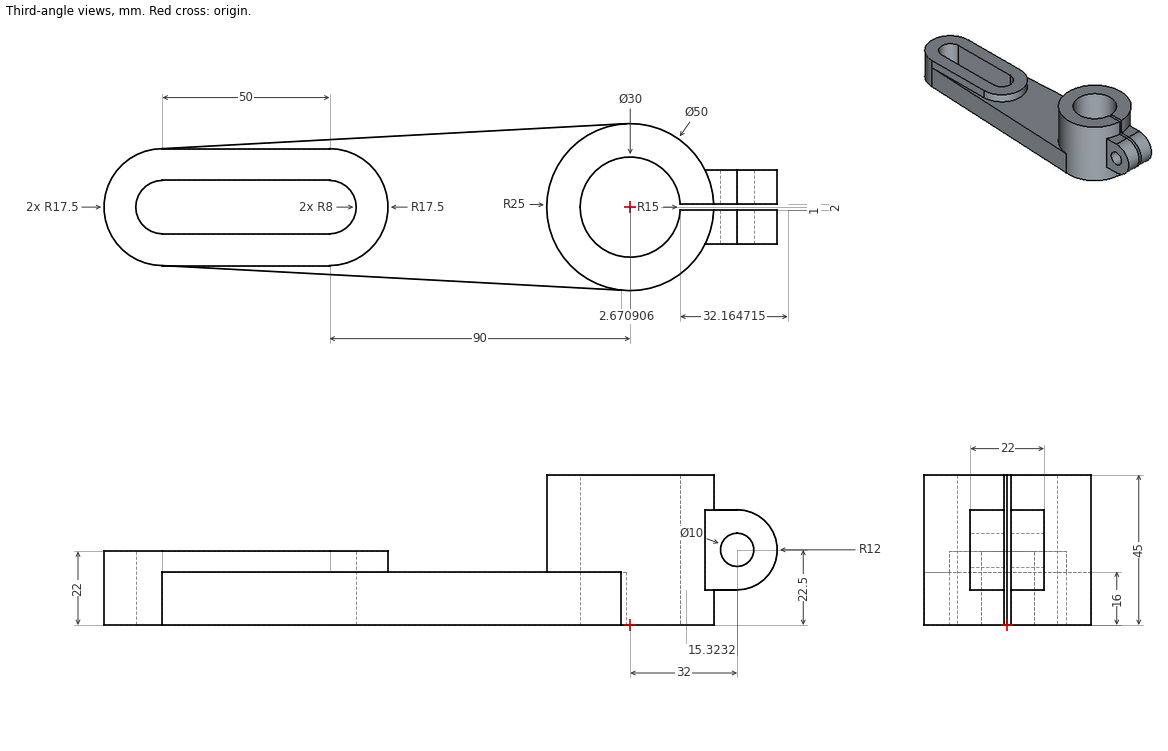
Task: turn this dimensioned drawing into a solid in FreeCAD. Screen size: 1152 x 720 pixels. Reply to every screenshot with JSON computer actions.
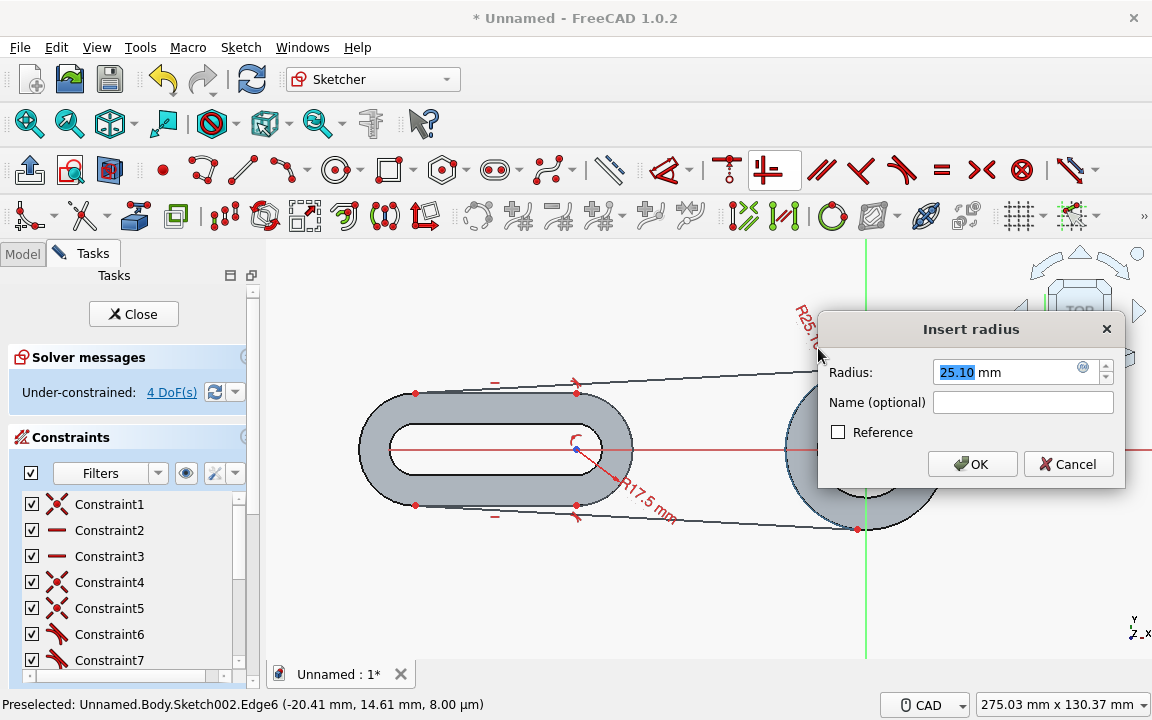
{"action": "type", "text": "25"}
{"action": "key", "text": "Return"}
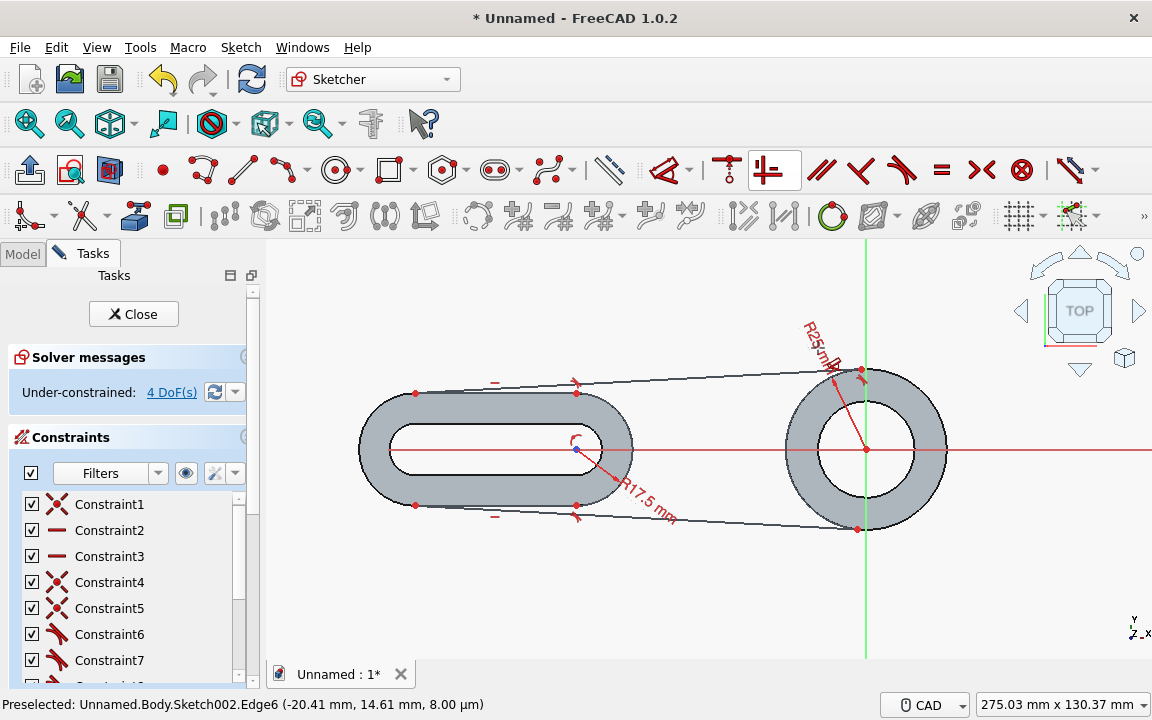
{"action": "scroll", "coordinate": [544, 393], "scroll_direction": "up", "scroll_amount": 4}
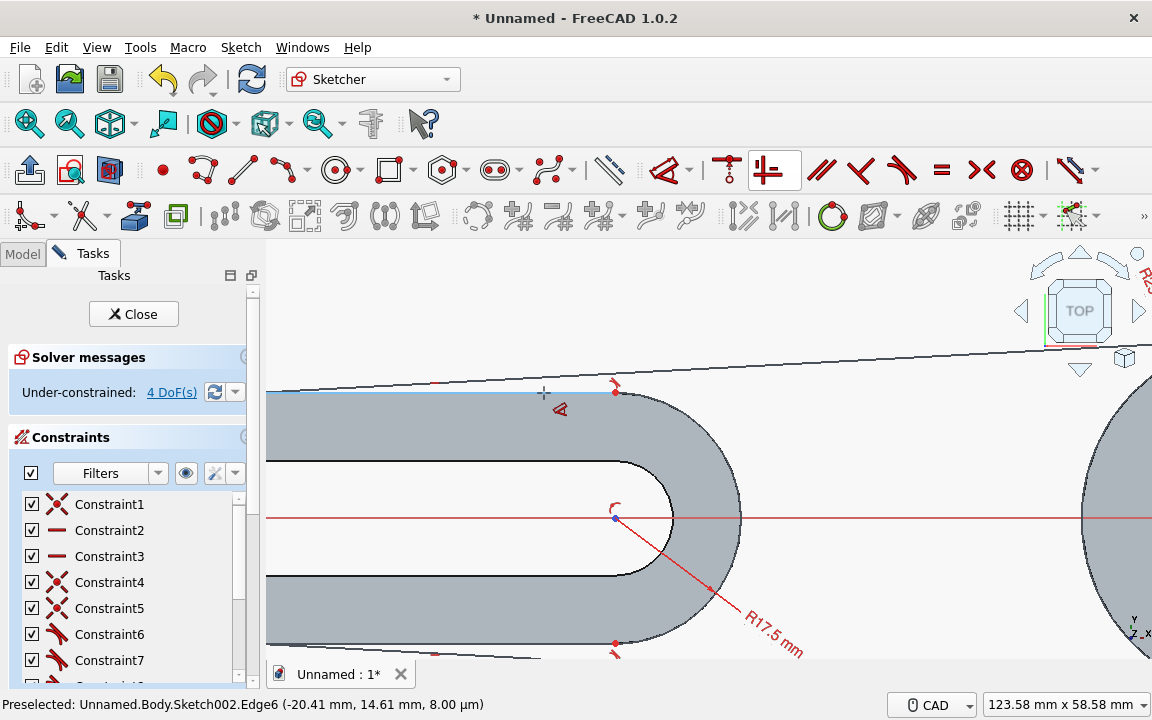
{"action": "left_click", "coordinate": [544, 393]}
{"action": "left_click", "coordinate": [455, 359]}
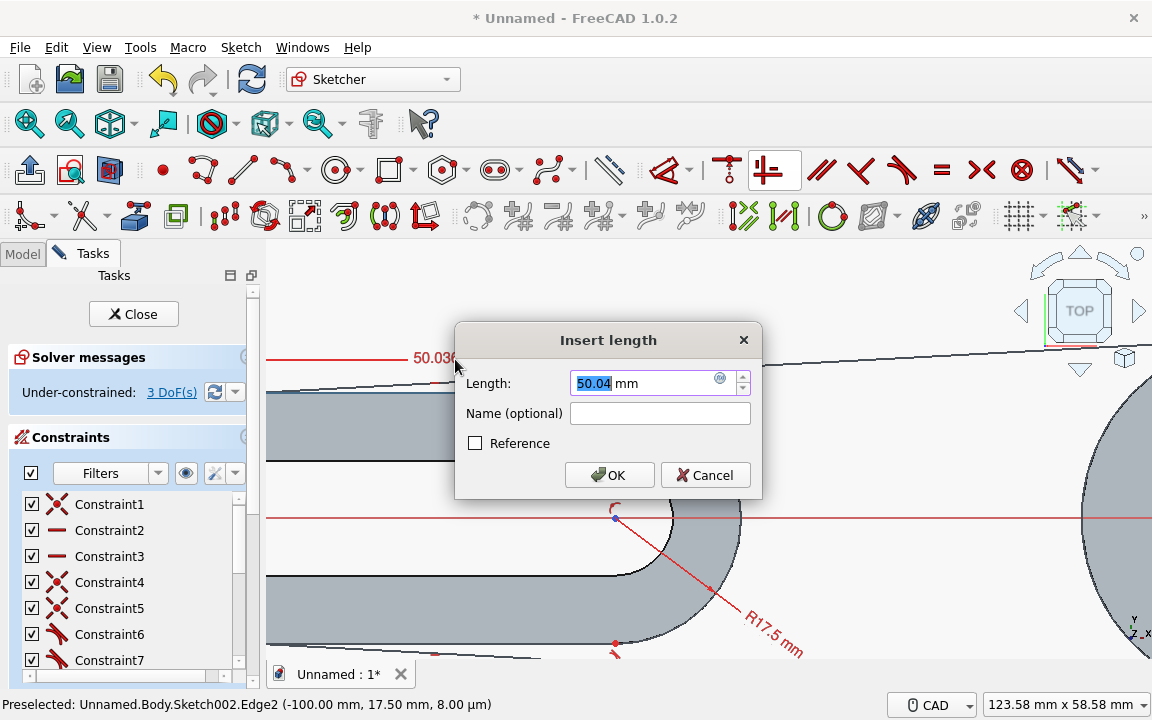
{"action": "type", "text": "50"}
{"action": "key", "text": "Return"}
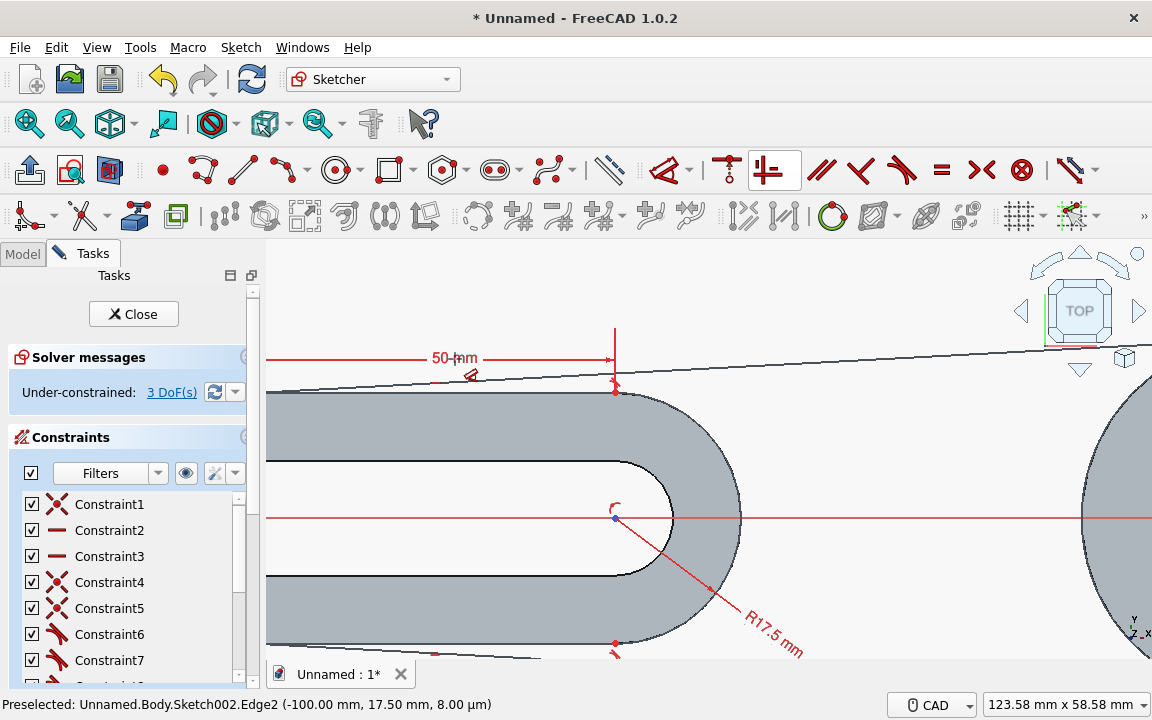
{"action": "scroll", "coordinate": [544, 393], "scroll_direction": "down", "scroll_amount": 4}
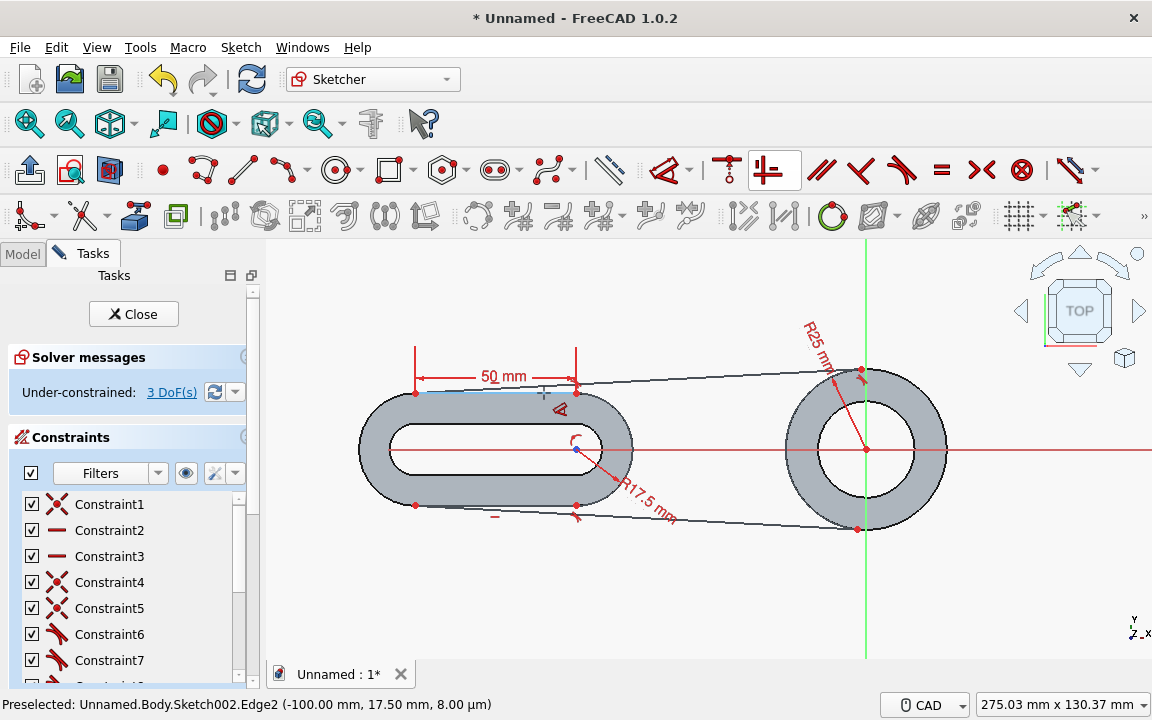
{"action": "scroll", "coordinate": [528, 506], "scroll_direction": "up", "scroll_amount": 5}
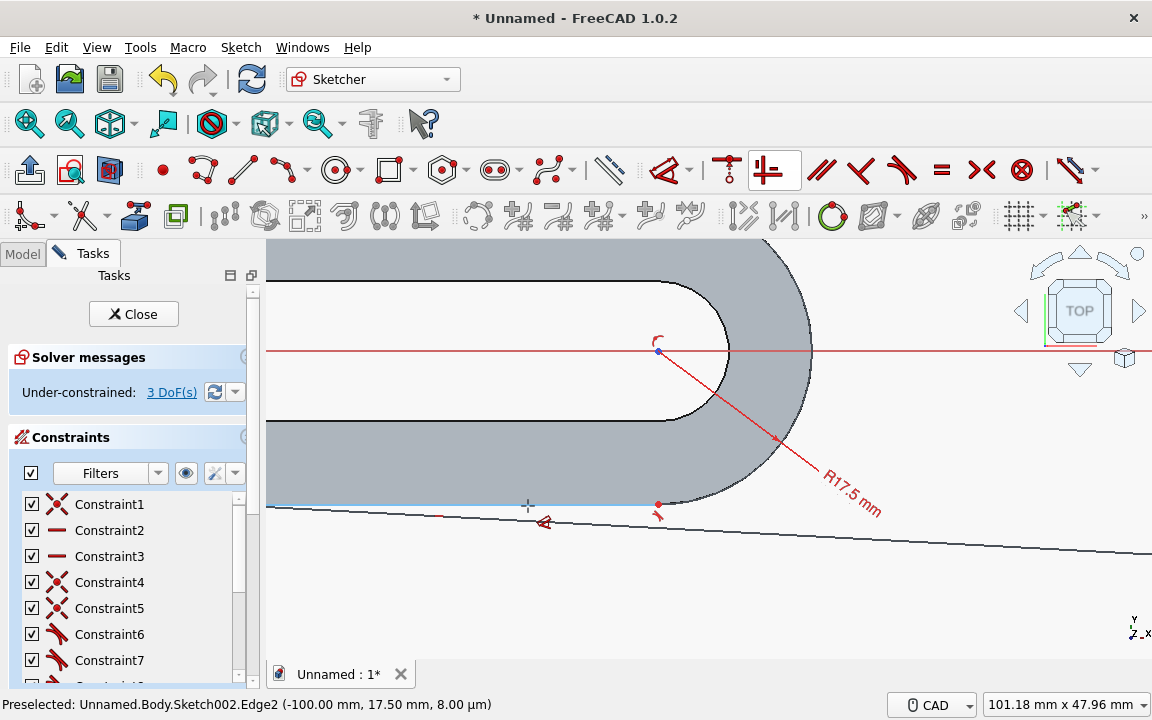
{"action": "left_click", "coordinate": [527, 505]}
{"action": "left_click", "coordinate": [476, 539]}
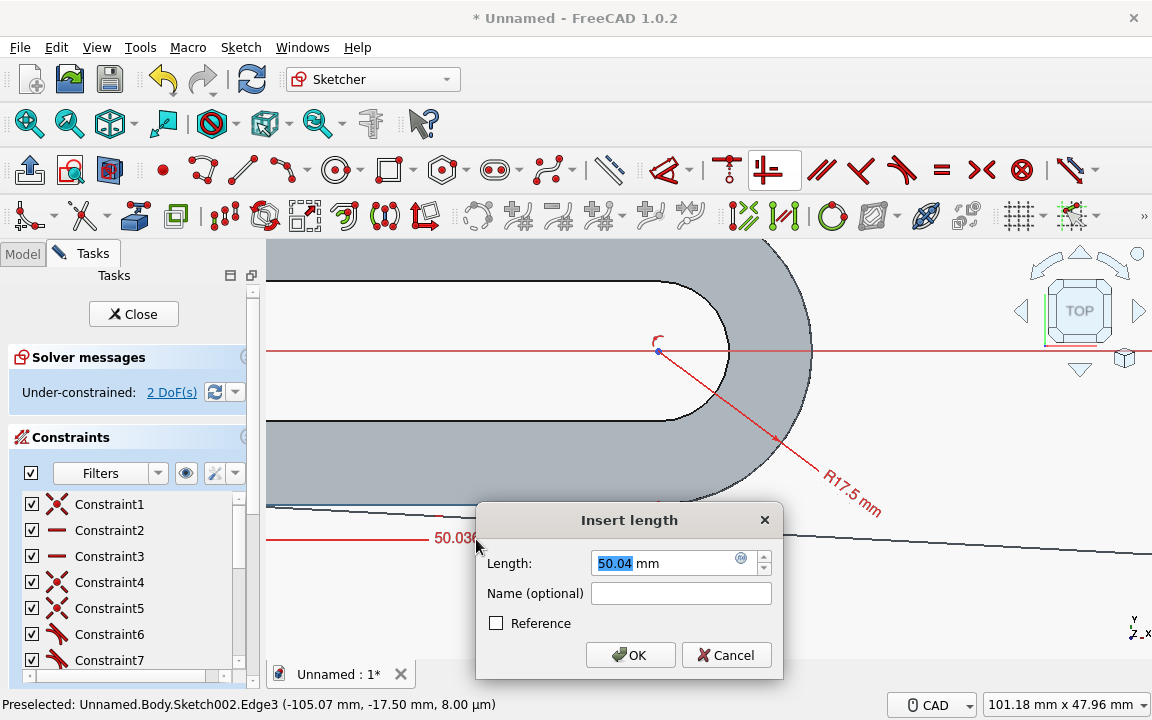
{"action": "type", "text": "50"}
{"action": "key", "text": "Return"}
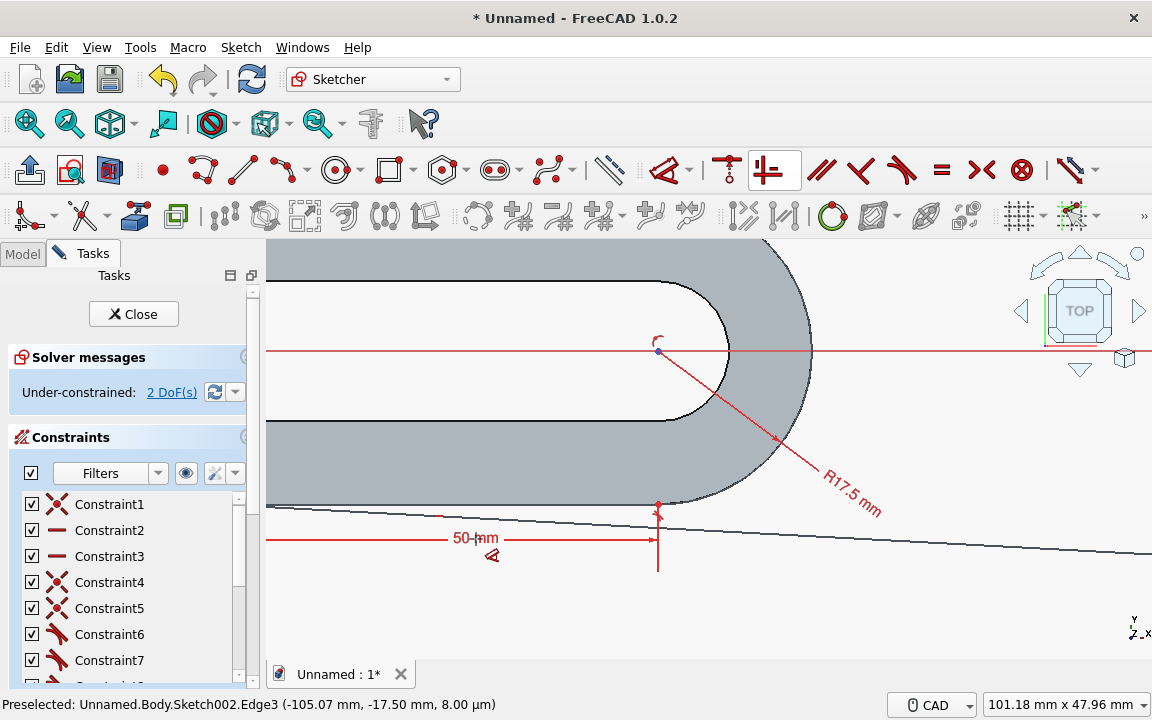
{"action": "scroll", "coordinate": [528, 506], "scroll_direction": "down", "scroll_amount": 5}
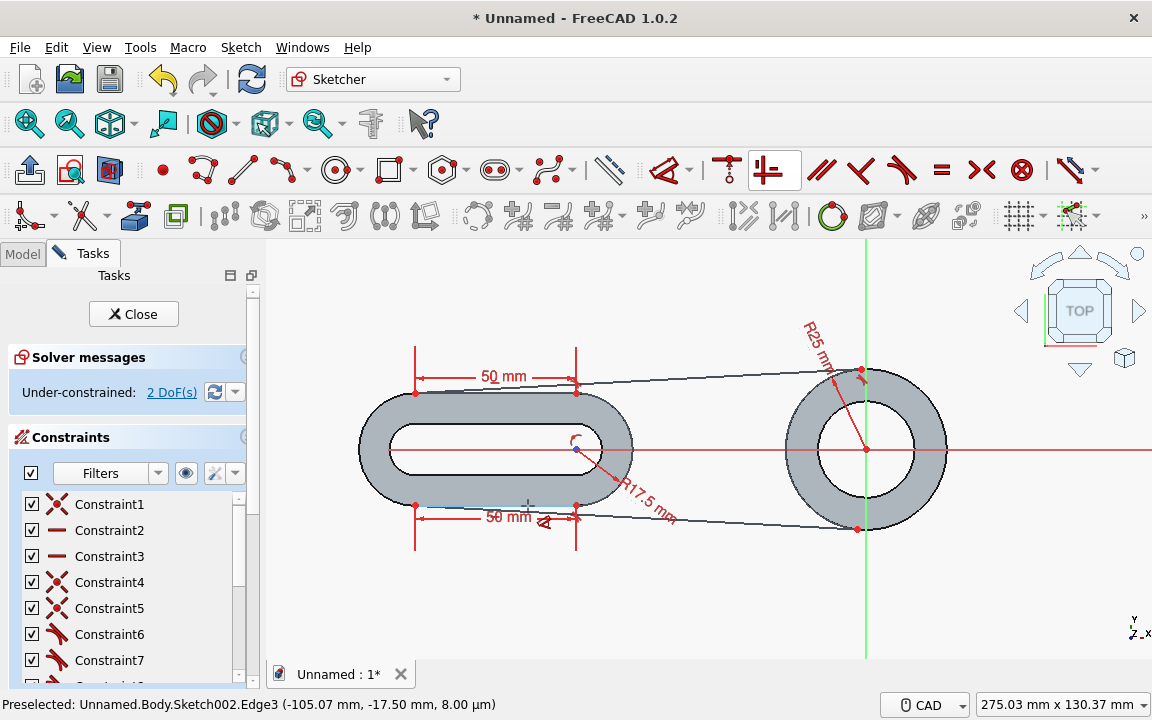
{"action": "left_click", "coordinate": [576, 393]}
{"action": "left_click", "coordinate": [721, 359]}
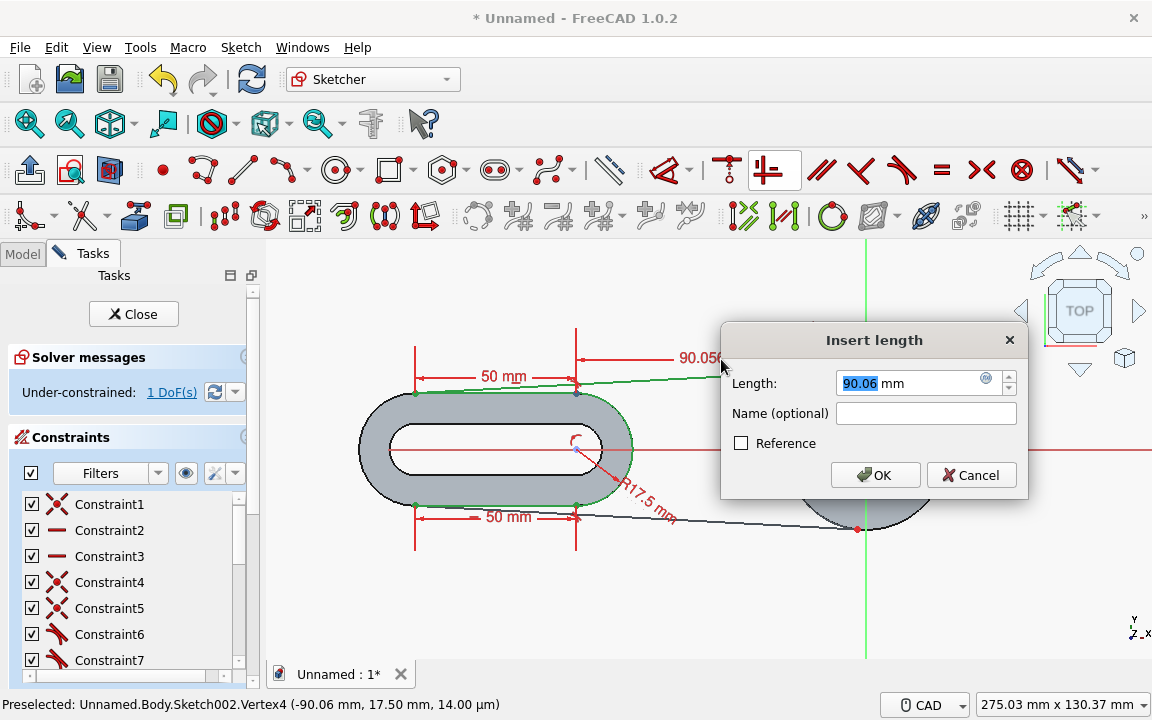
{"action": "type", "text": "90"}
{"action": "key", "text": "Return"}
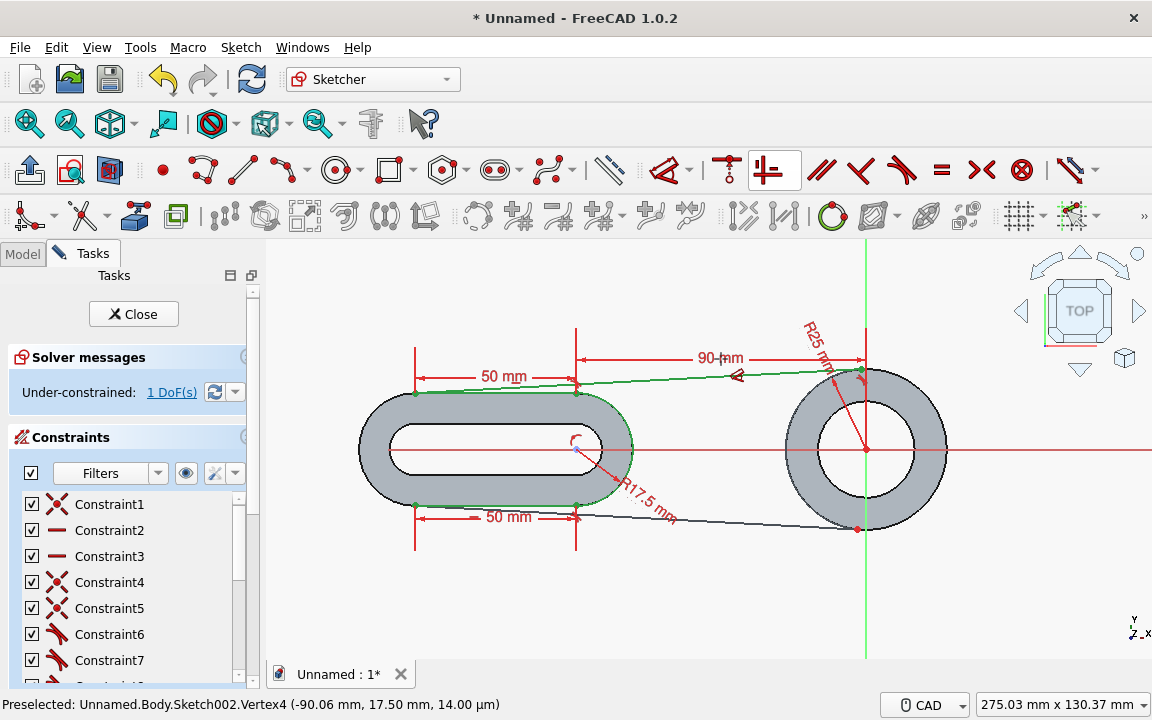
{"action": "scroll", "coordinate": [858, 530], "scroll_direction": "up", "scroll_amount": 8}